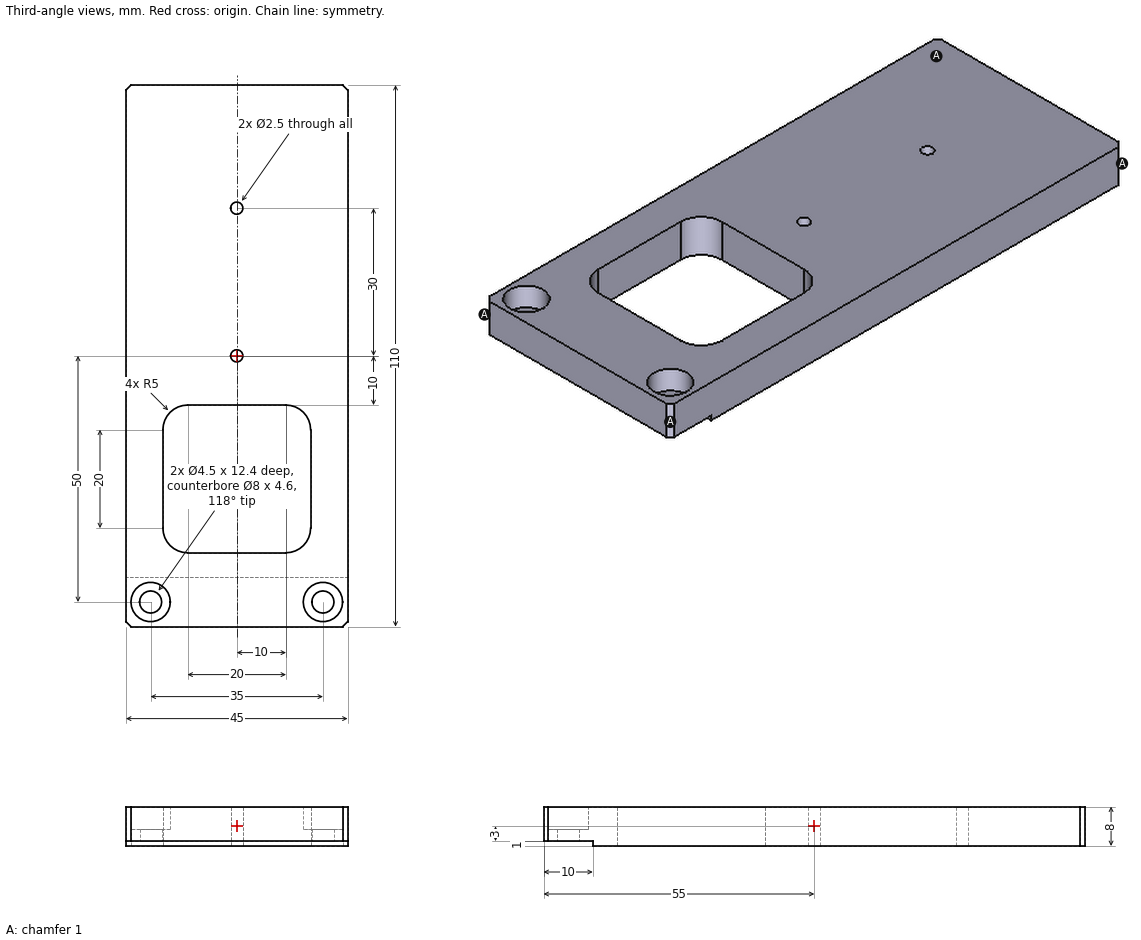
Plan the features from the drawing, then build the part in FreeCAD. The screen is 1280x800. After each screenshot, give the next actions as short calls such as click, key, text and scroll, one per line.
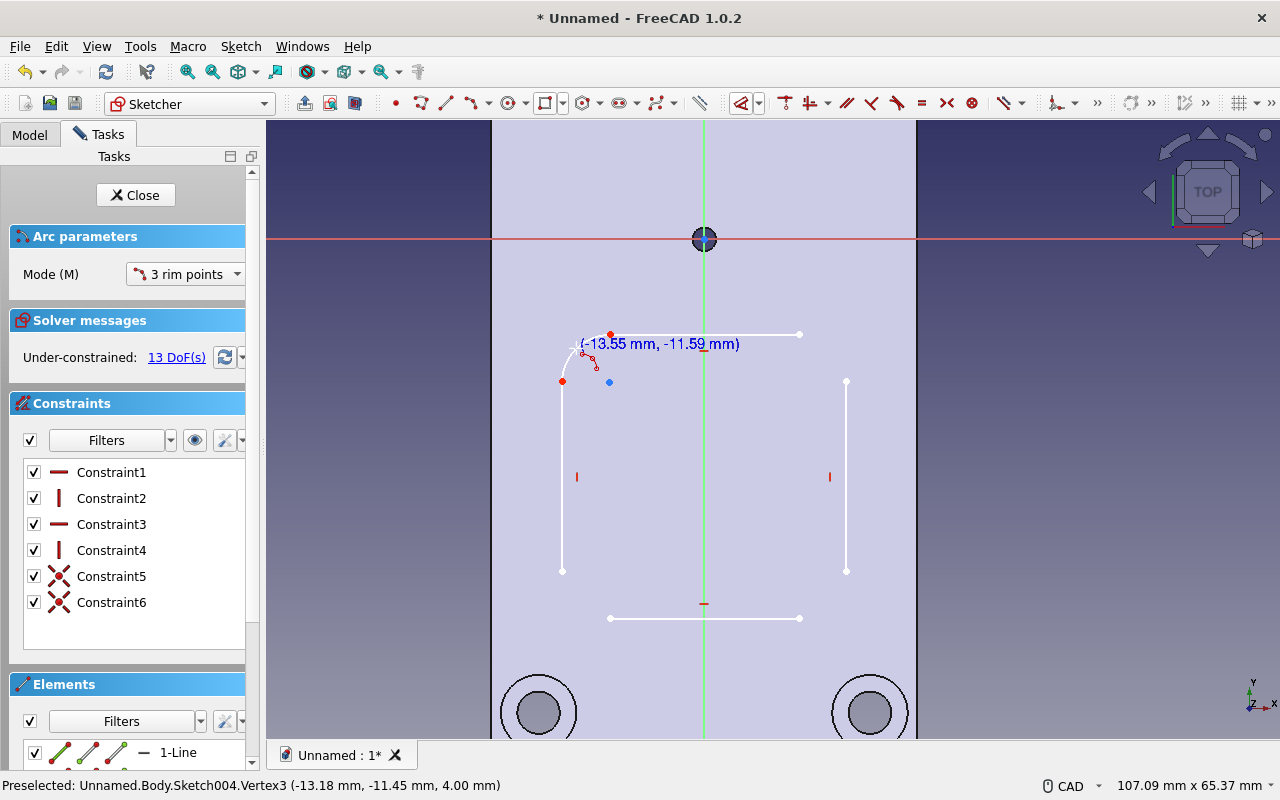
click(562, 572)
click(610, 619)
click(576, 604)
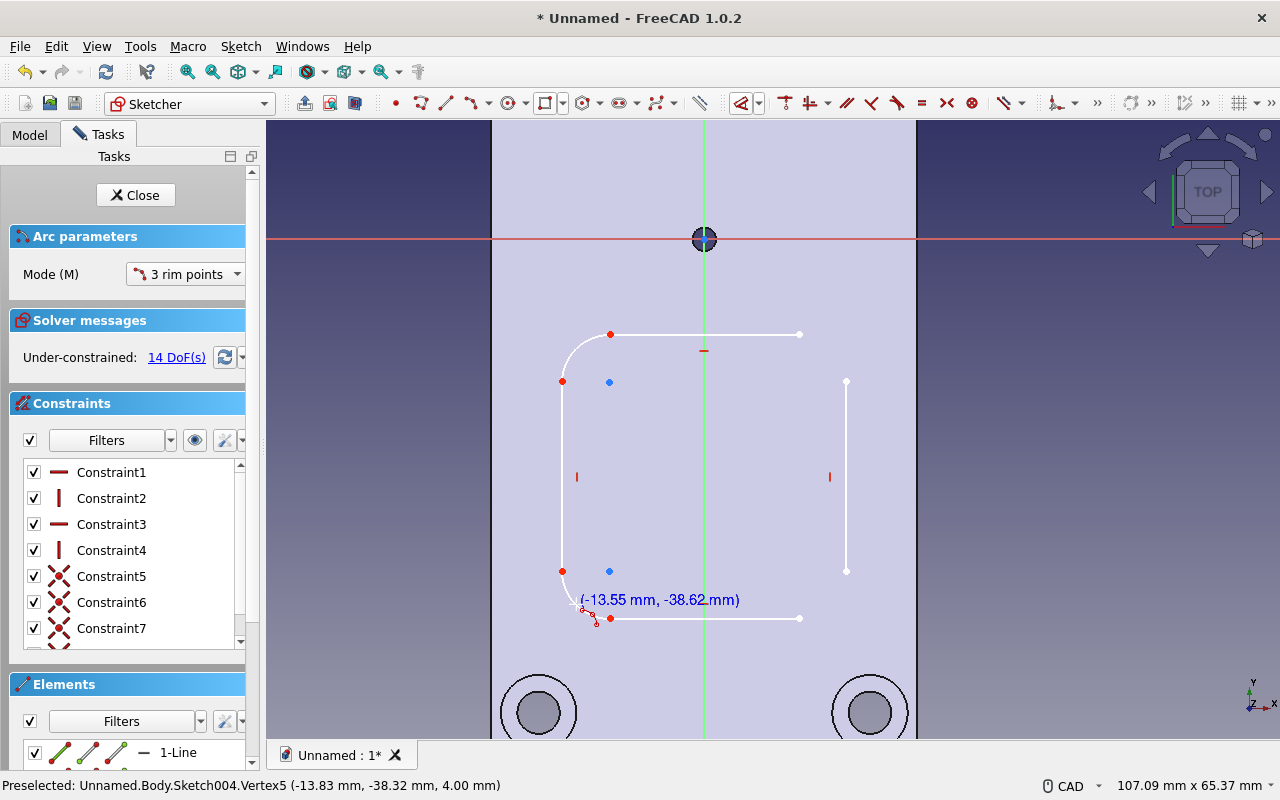
click(799, 619)
click(846, 572)
click(832, 604)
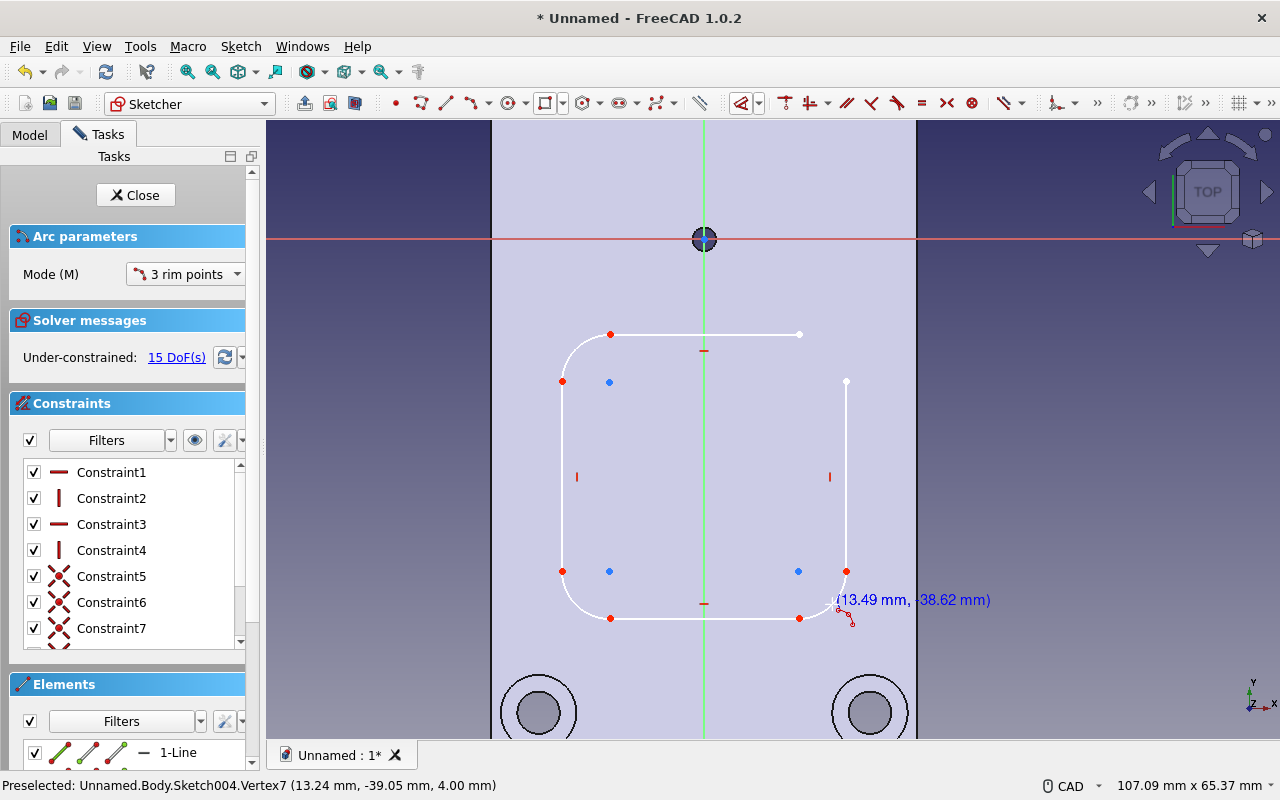
click(846, 382)
click(799, 335)
click(832, 348)
key(Escape)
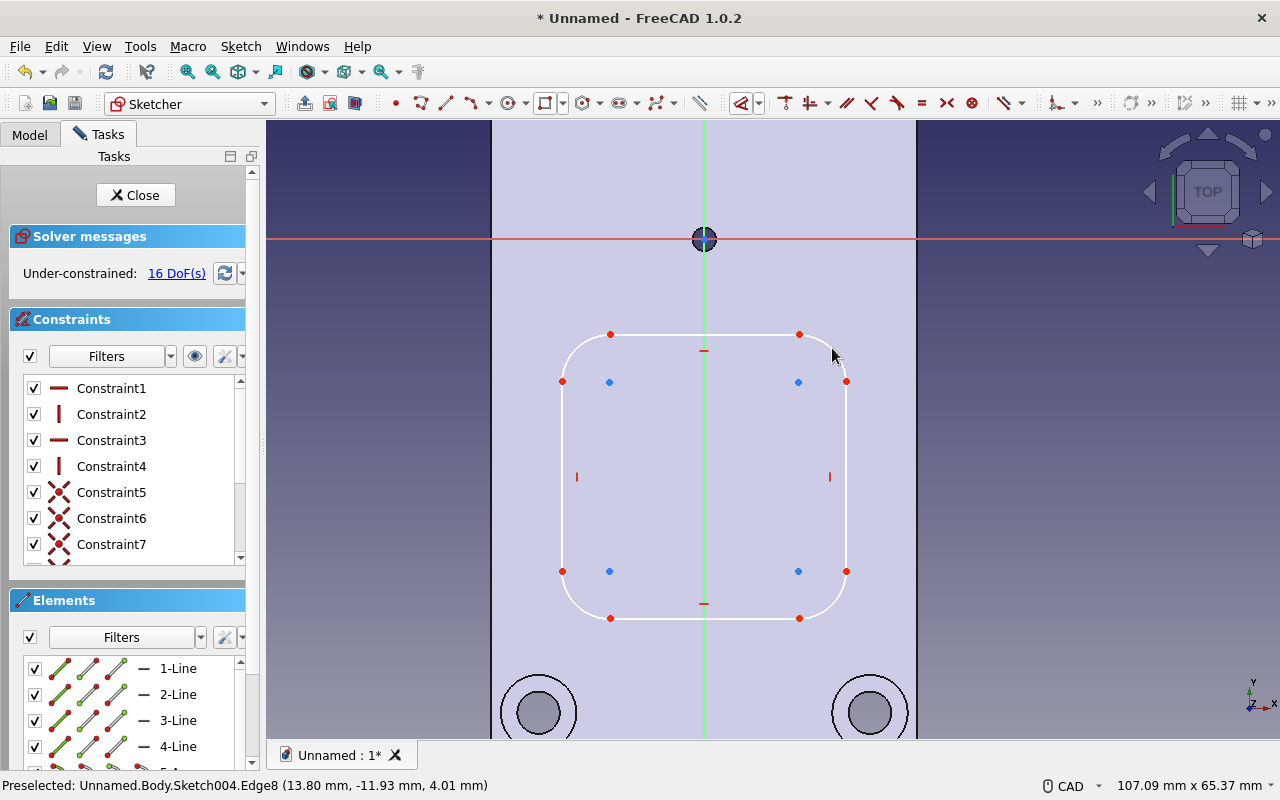
click(742, 335)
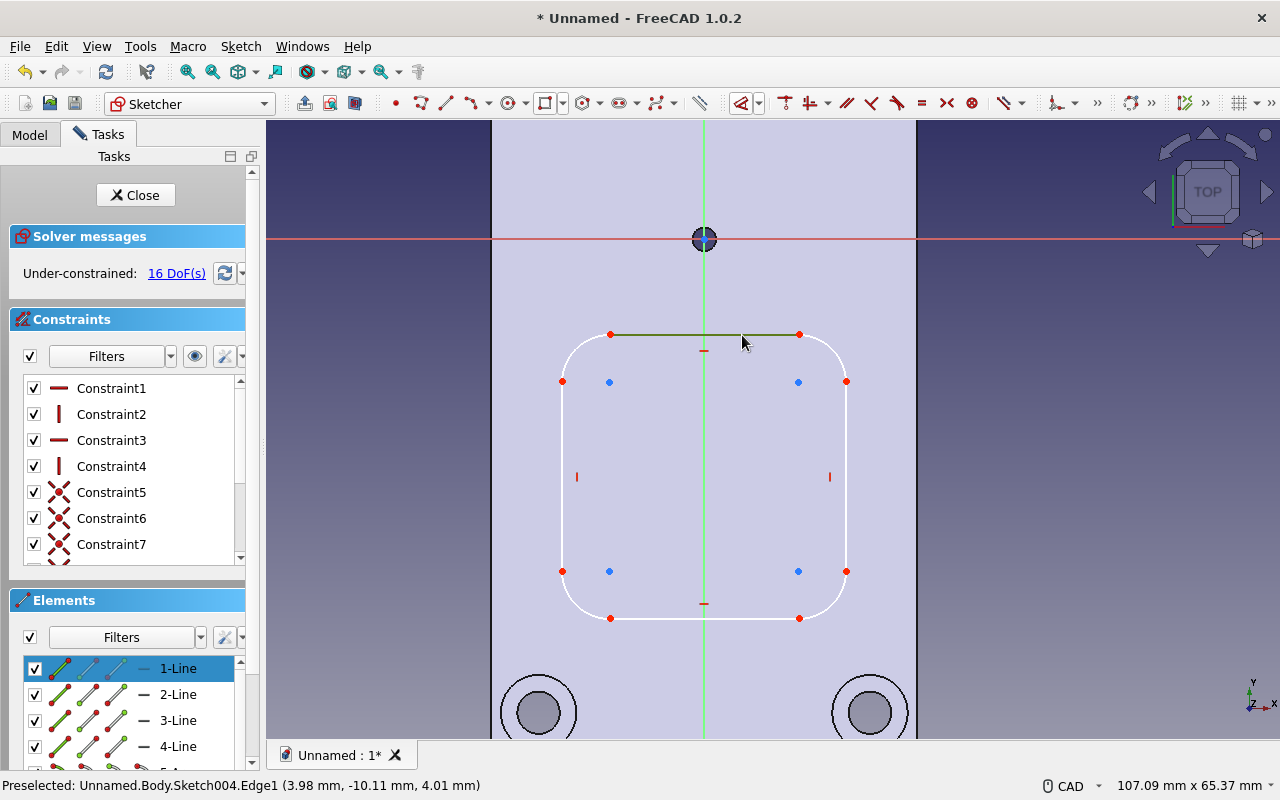
click(588, 340)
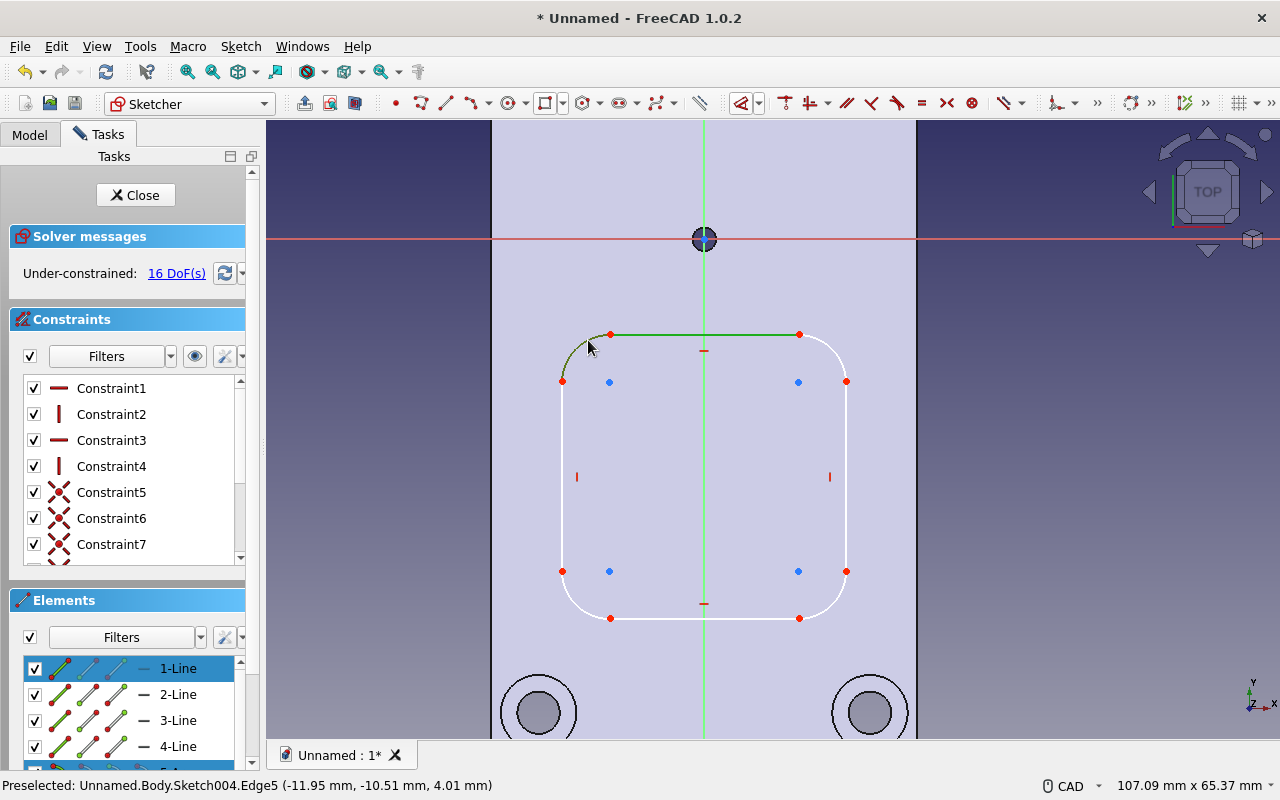
click(897, 104)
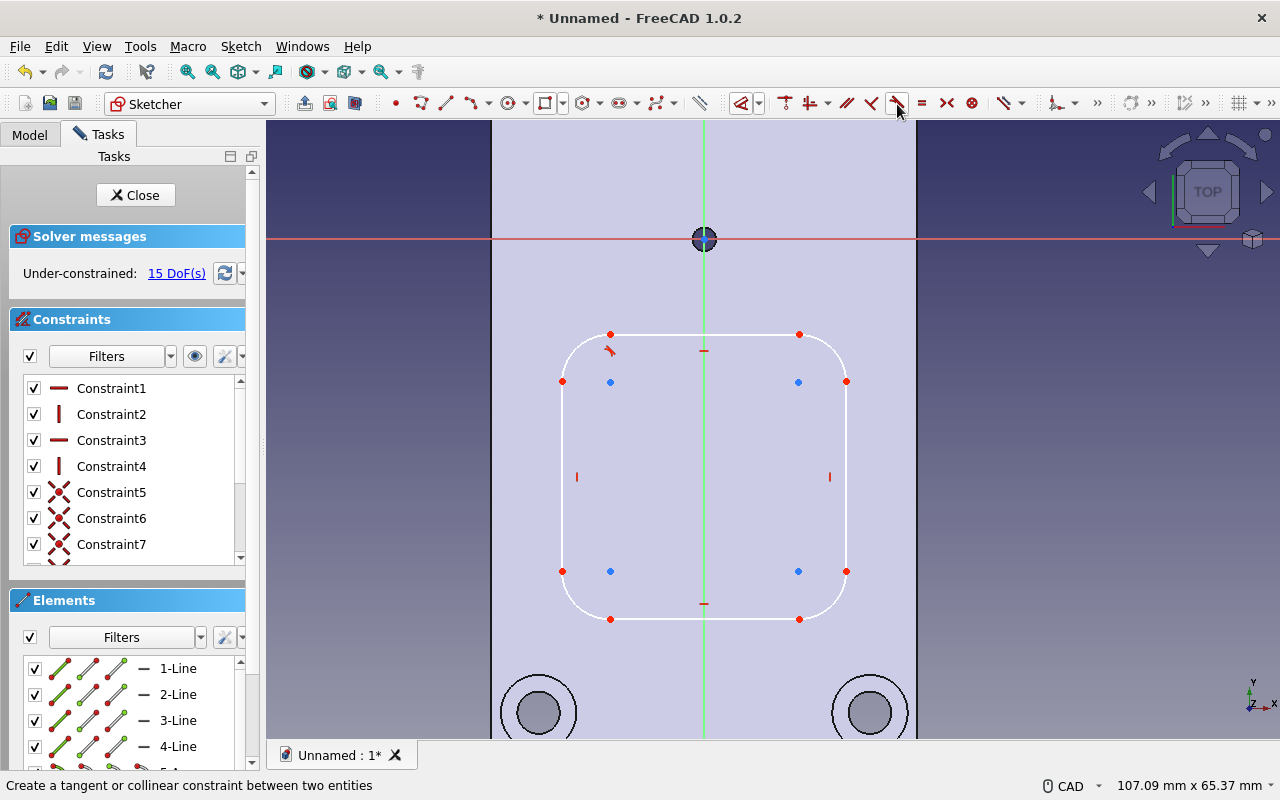
click(742, 335)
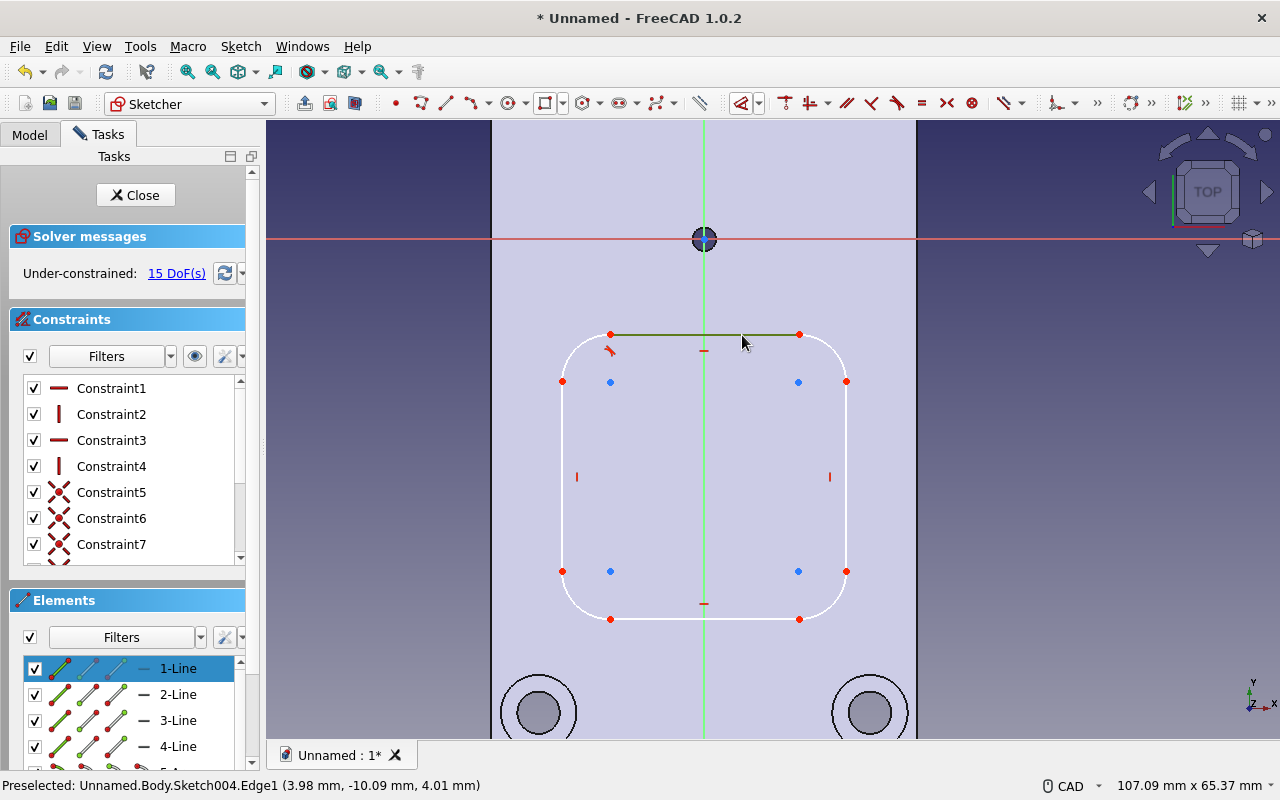
click(841, 361)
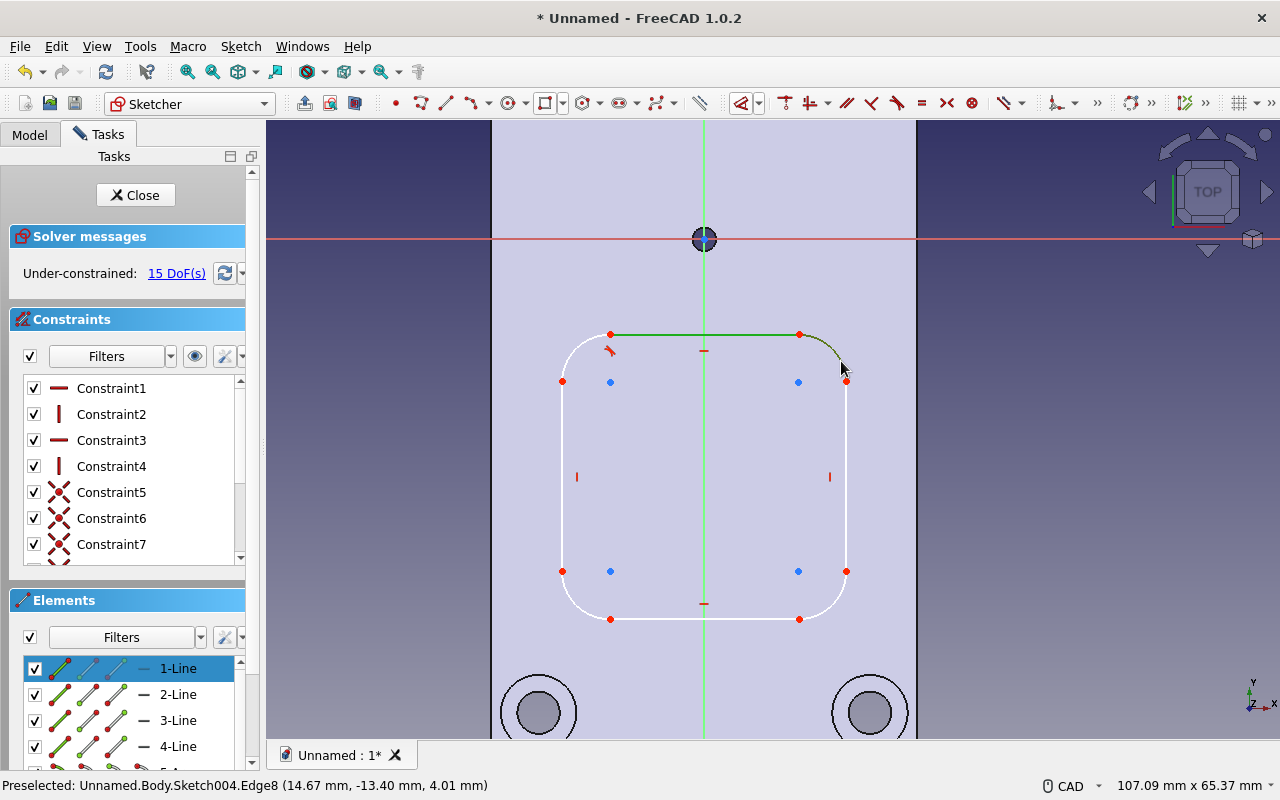
click(897, 104)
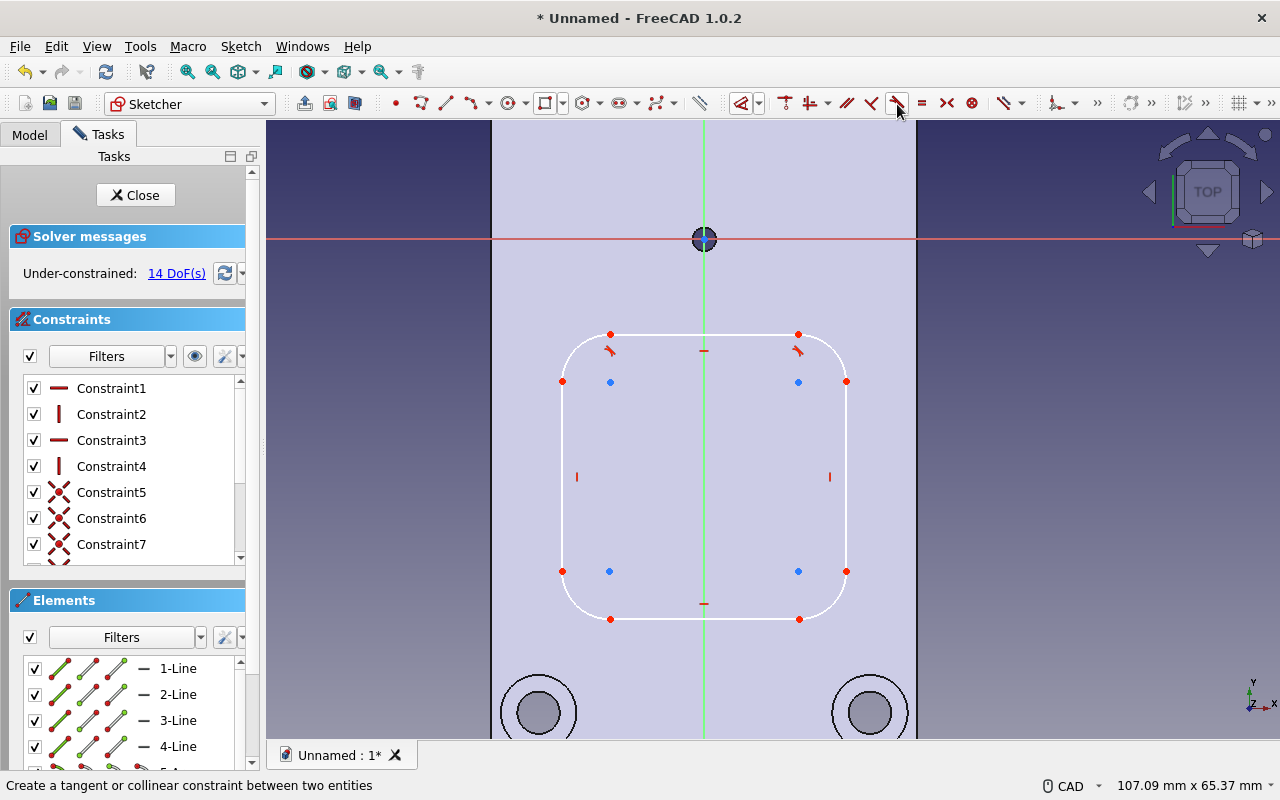
click(562, 439)